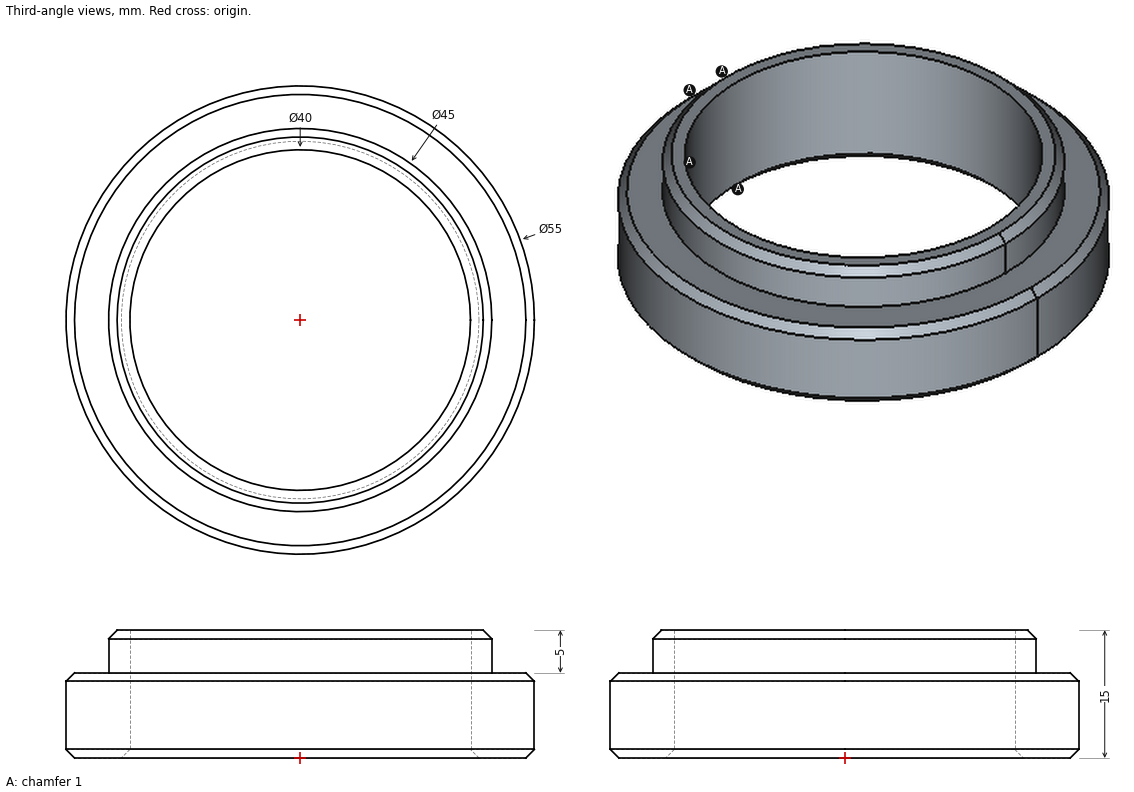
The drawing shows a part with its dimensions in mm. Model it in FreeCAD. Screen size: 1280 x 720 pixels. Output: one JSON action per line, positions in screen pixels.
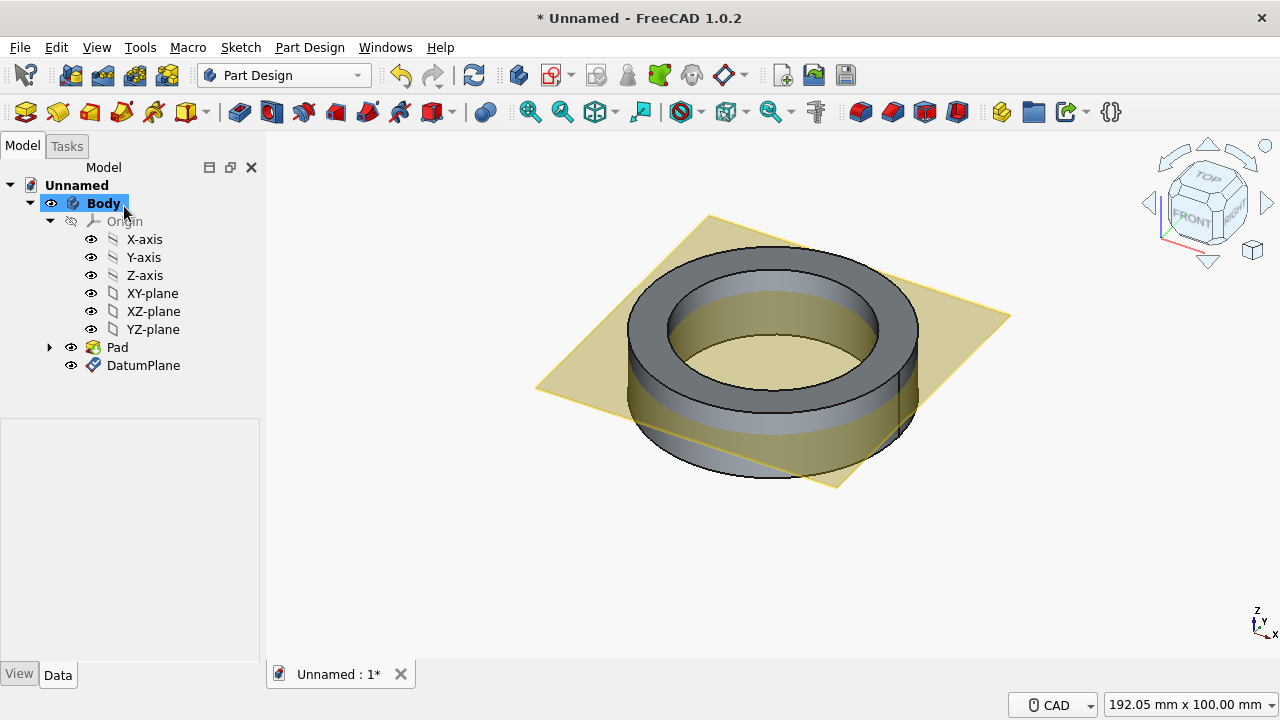
{"action": "left_click", "coordinate": [116, 365]}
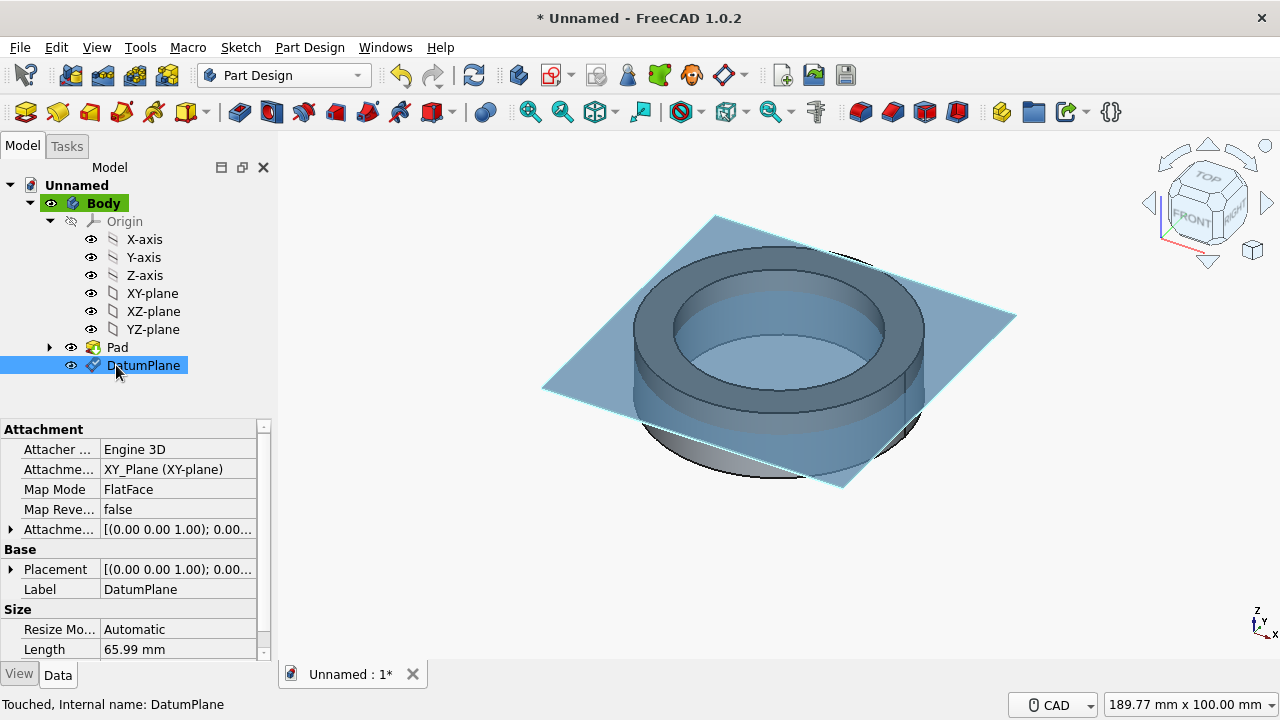
{"action": "left_click", "coordinate": [552, 76]}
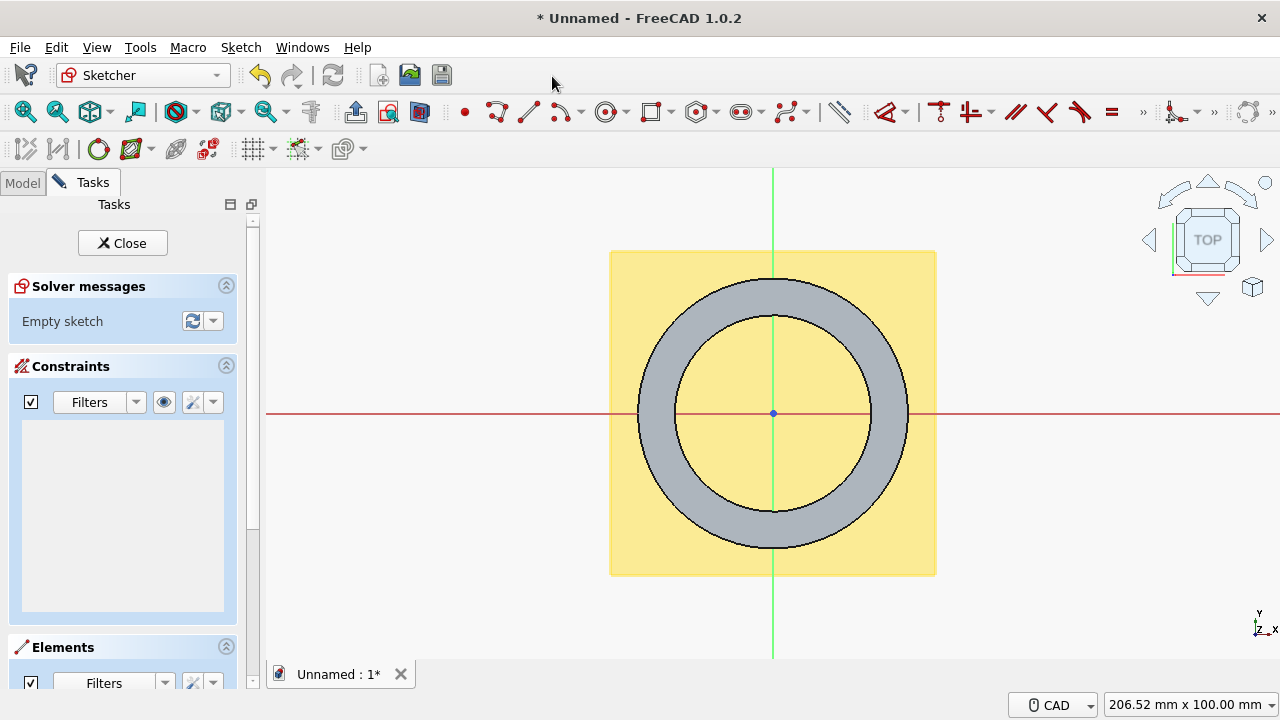
{"action": "key", "text": "q s"}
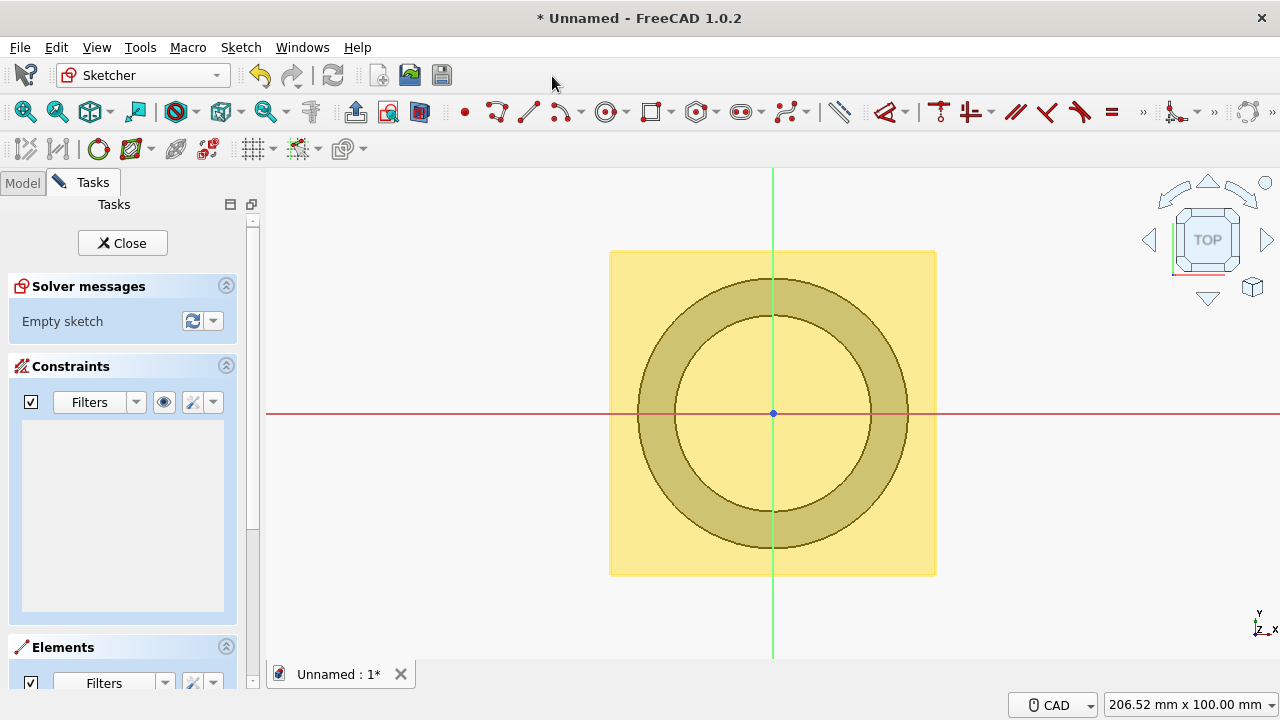
{"action": "left_click", "coordinate": [606, 112]}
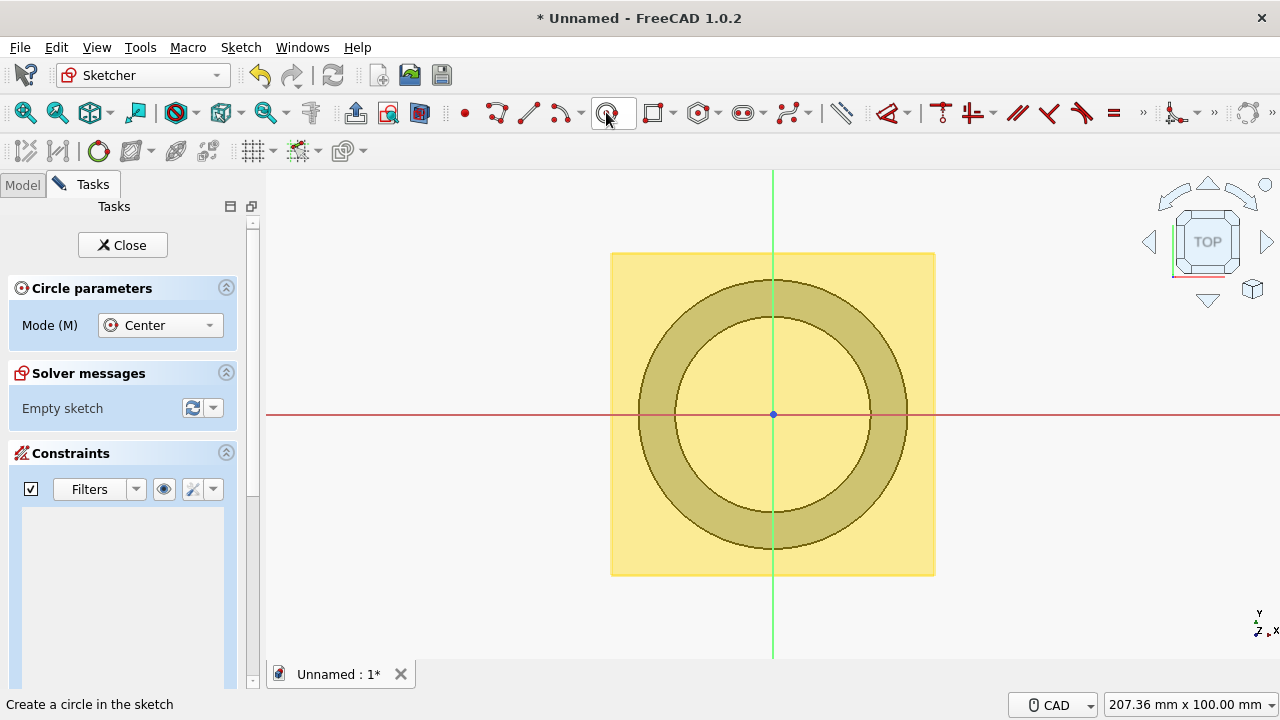
{"action": "left_click", "coordinate": [773, 414]}
{"action": "mouse_move", "coordinate": [868, 319]}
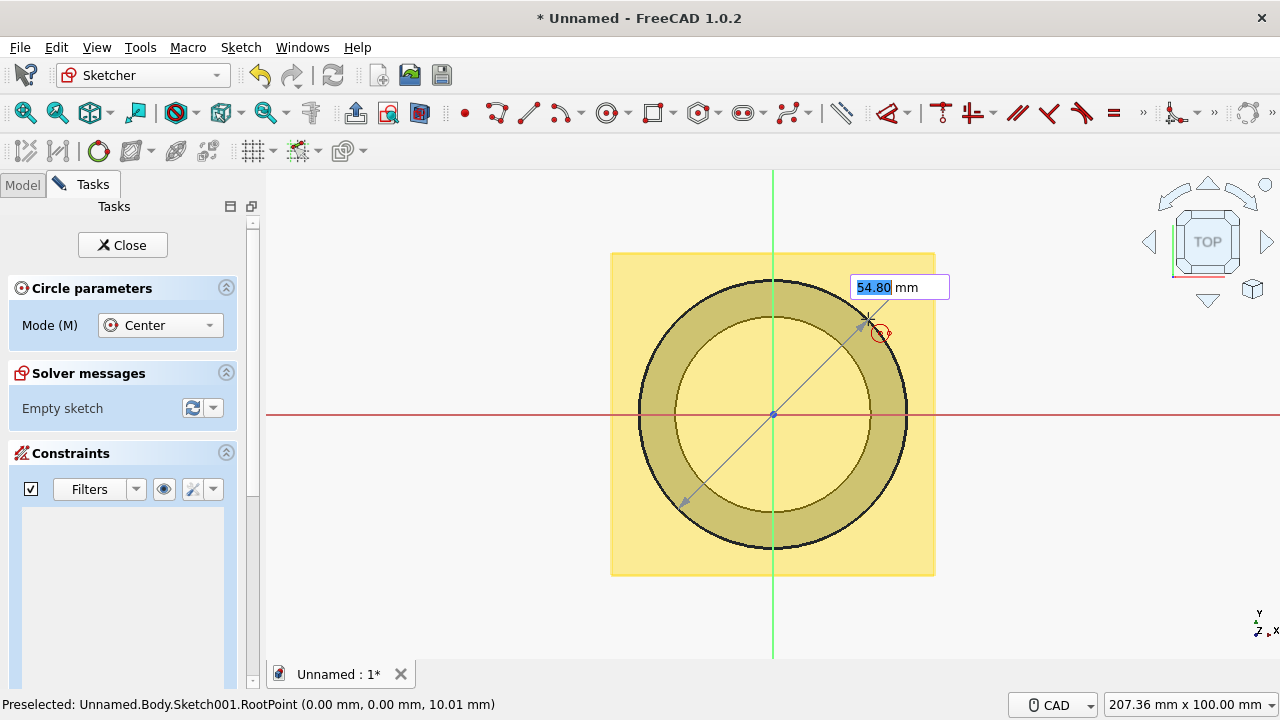
{"action": "type", "text": "55"}
{"action": "key", "text": "Return"}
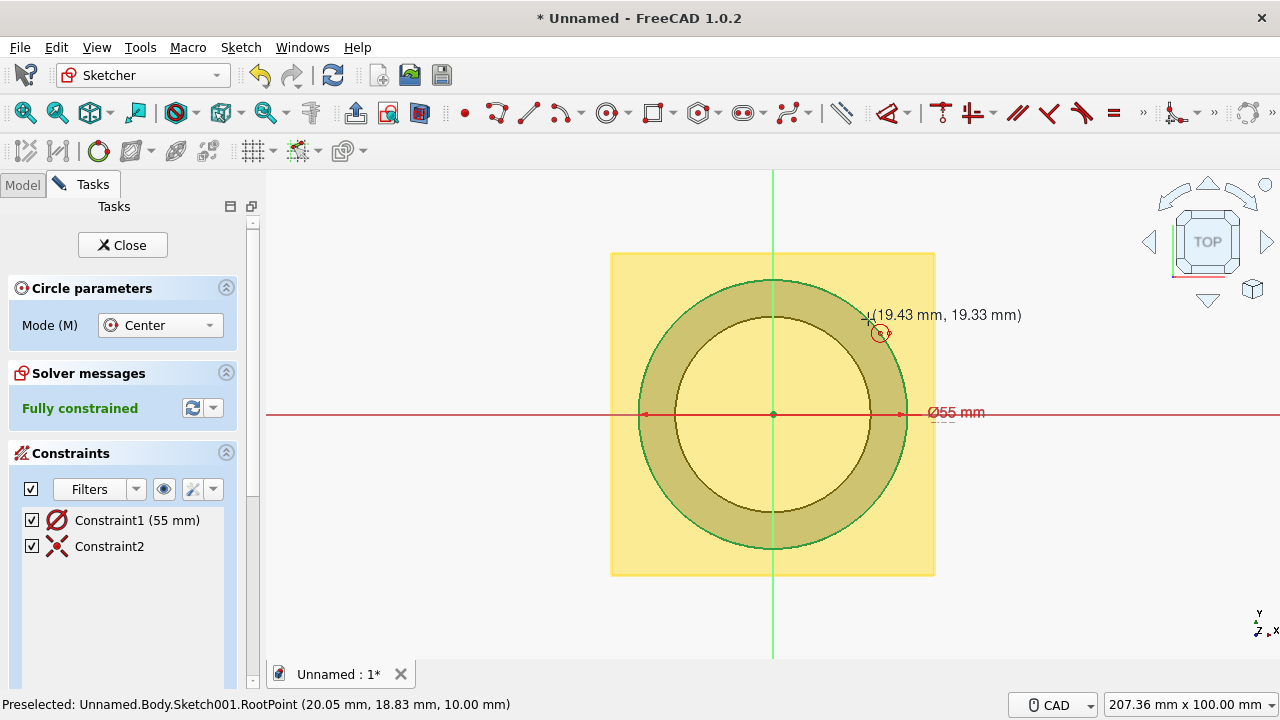
{"action": "left_click", "coordinate": [773, 414]}
{"action": "mouse_move", "coordinate": [851, 337]}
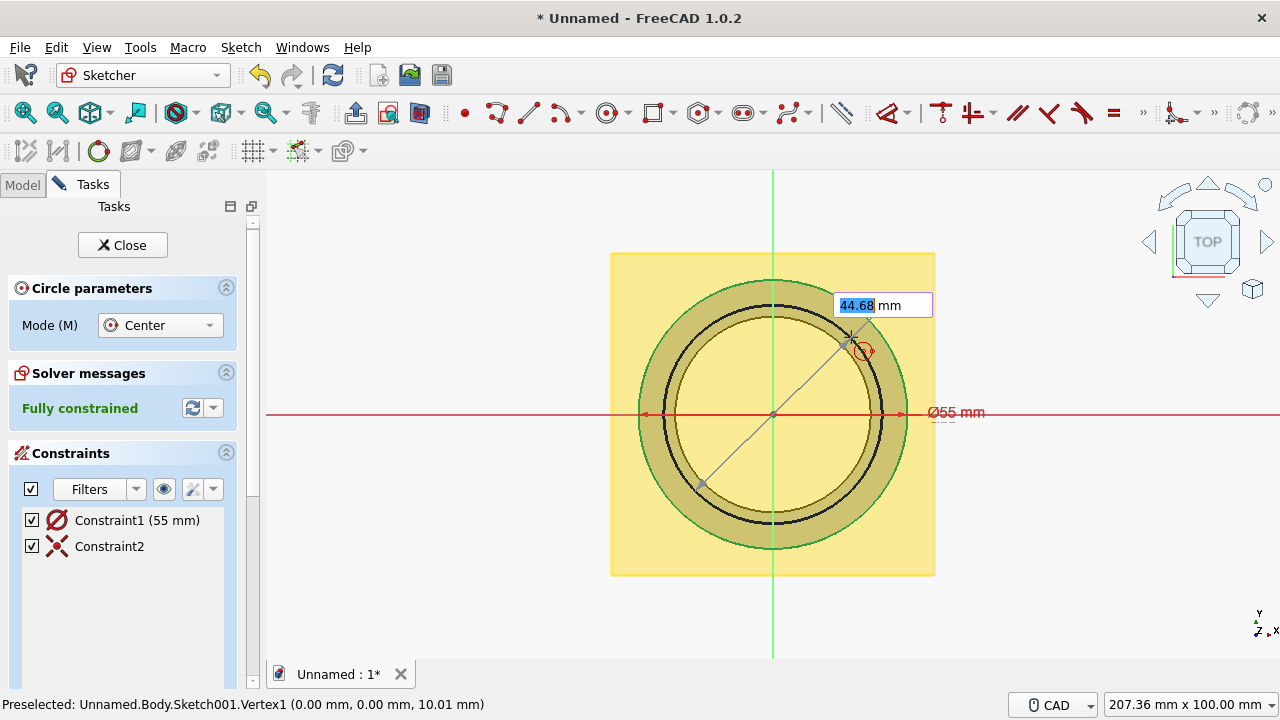
{"action": "type", "text": "45"}
{"action": "key", "text": "Return"}
{"action": "key", "text": "Escape"}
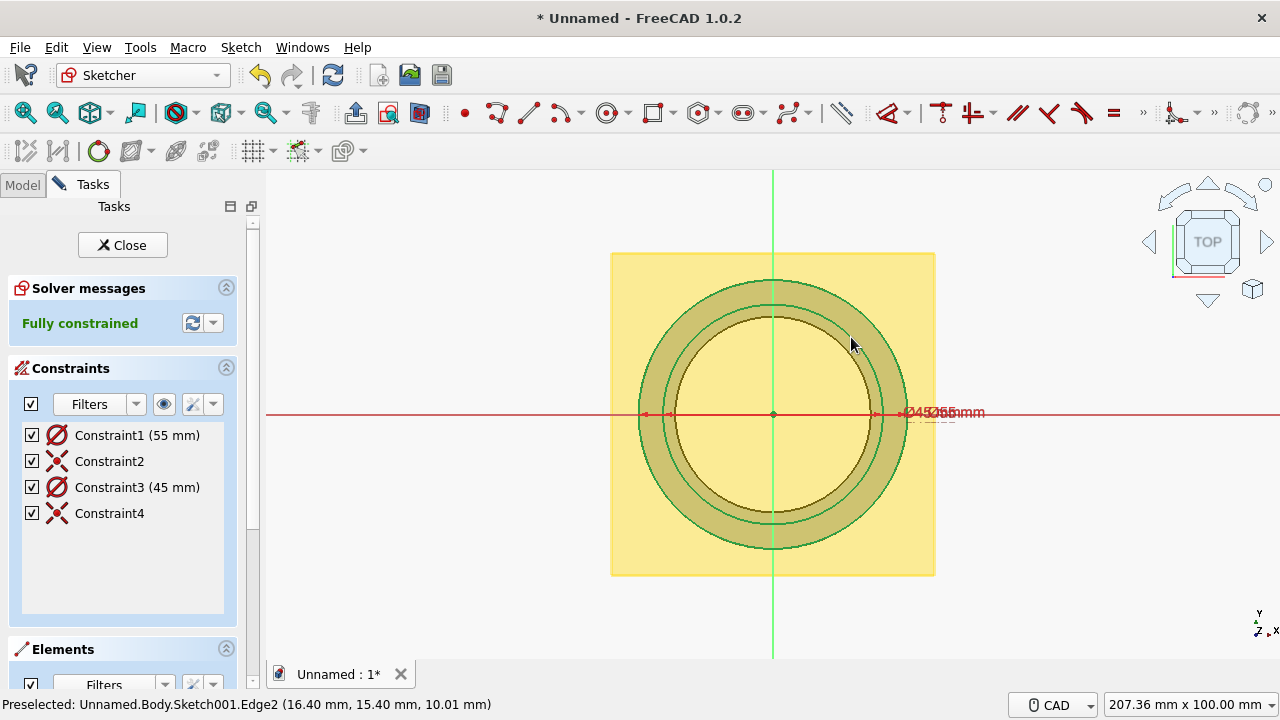
{"action": "left_click", "coordinate": [123, 245]}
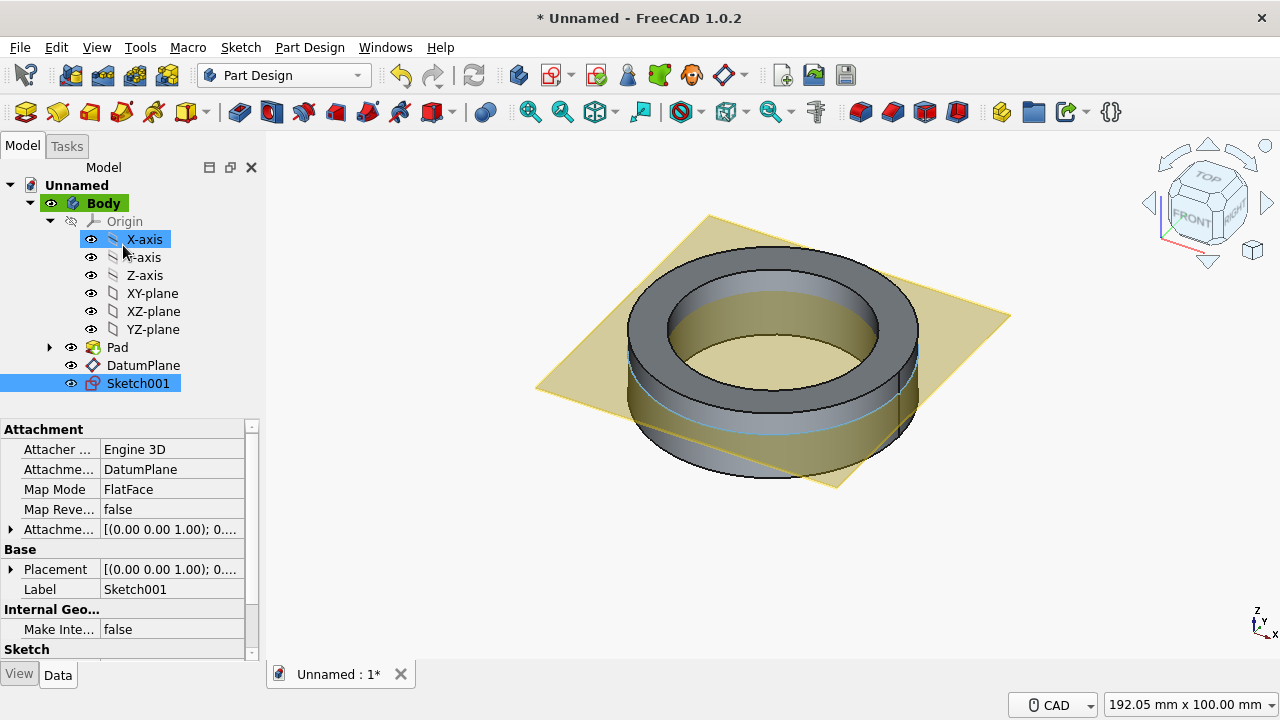
{"action": "left_click", "coordinate": [240, 112]}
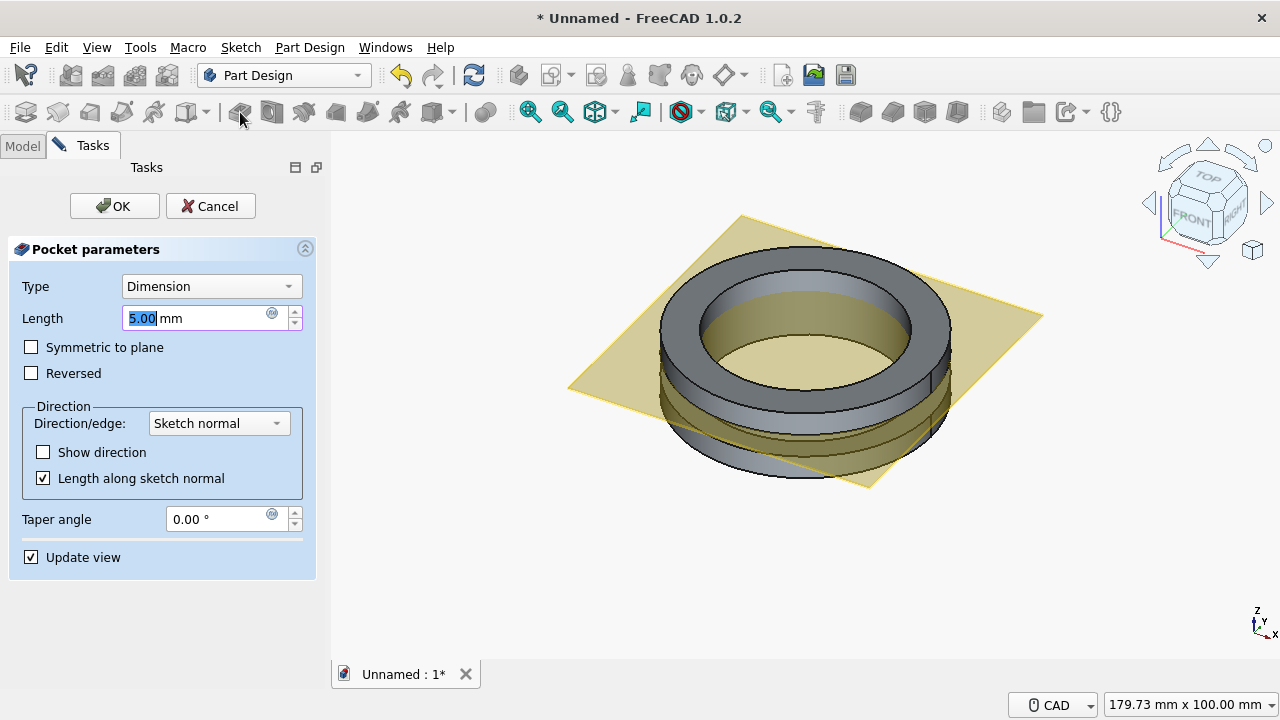
{"action": "type", "text": "5"}
{"action": "key", "text": "Tab"}